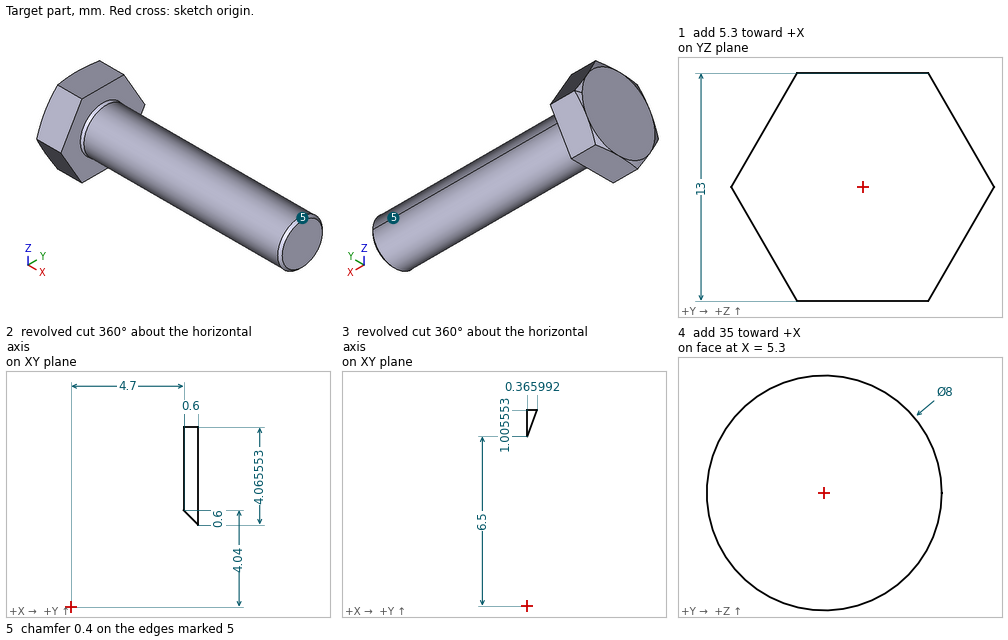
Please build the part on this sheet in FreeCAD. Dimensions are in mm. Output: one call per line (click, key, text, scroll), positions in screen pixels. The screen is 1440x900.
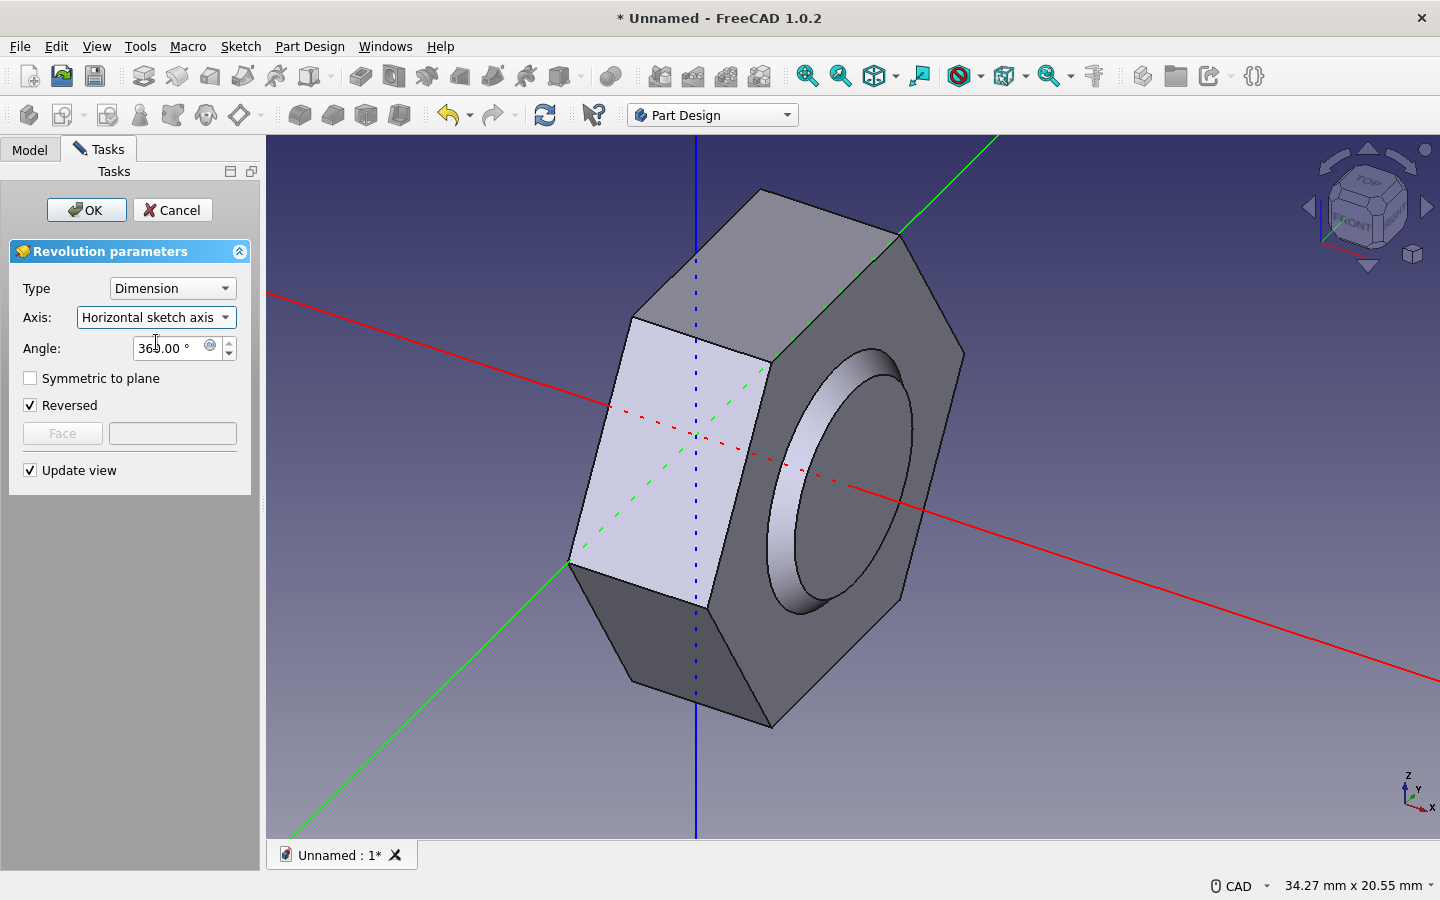
click(87, 210)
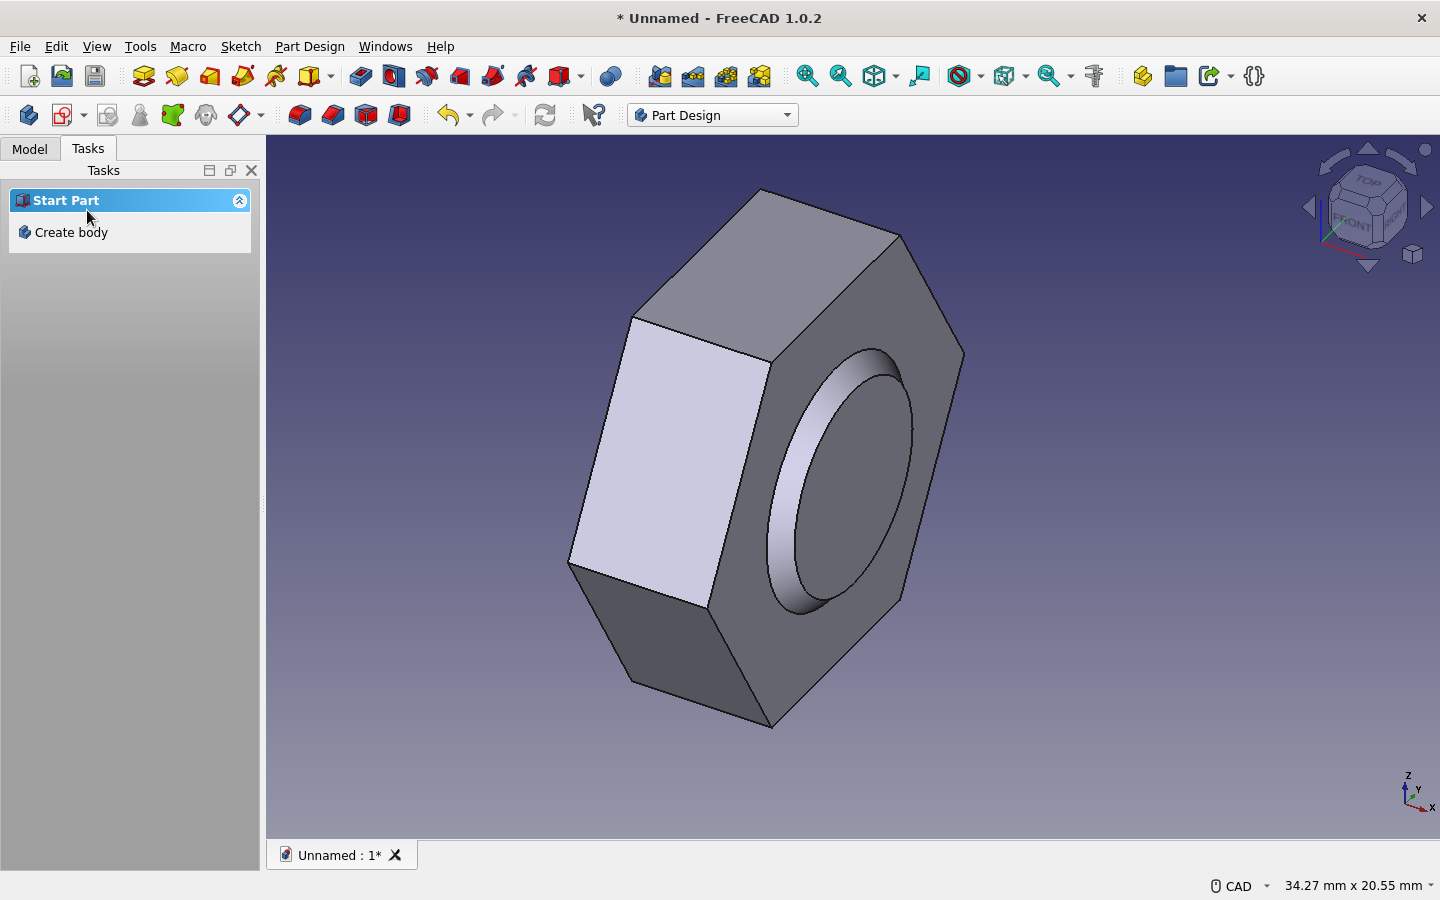
key(v)
key(f)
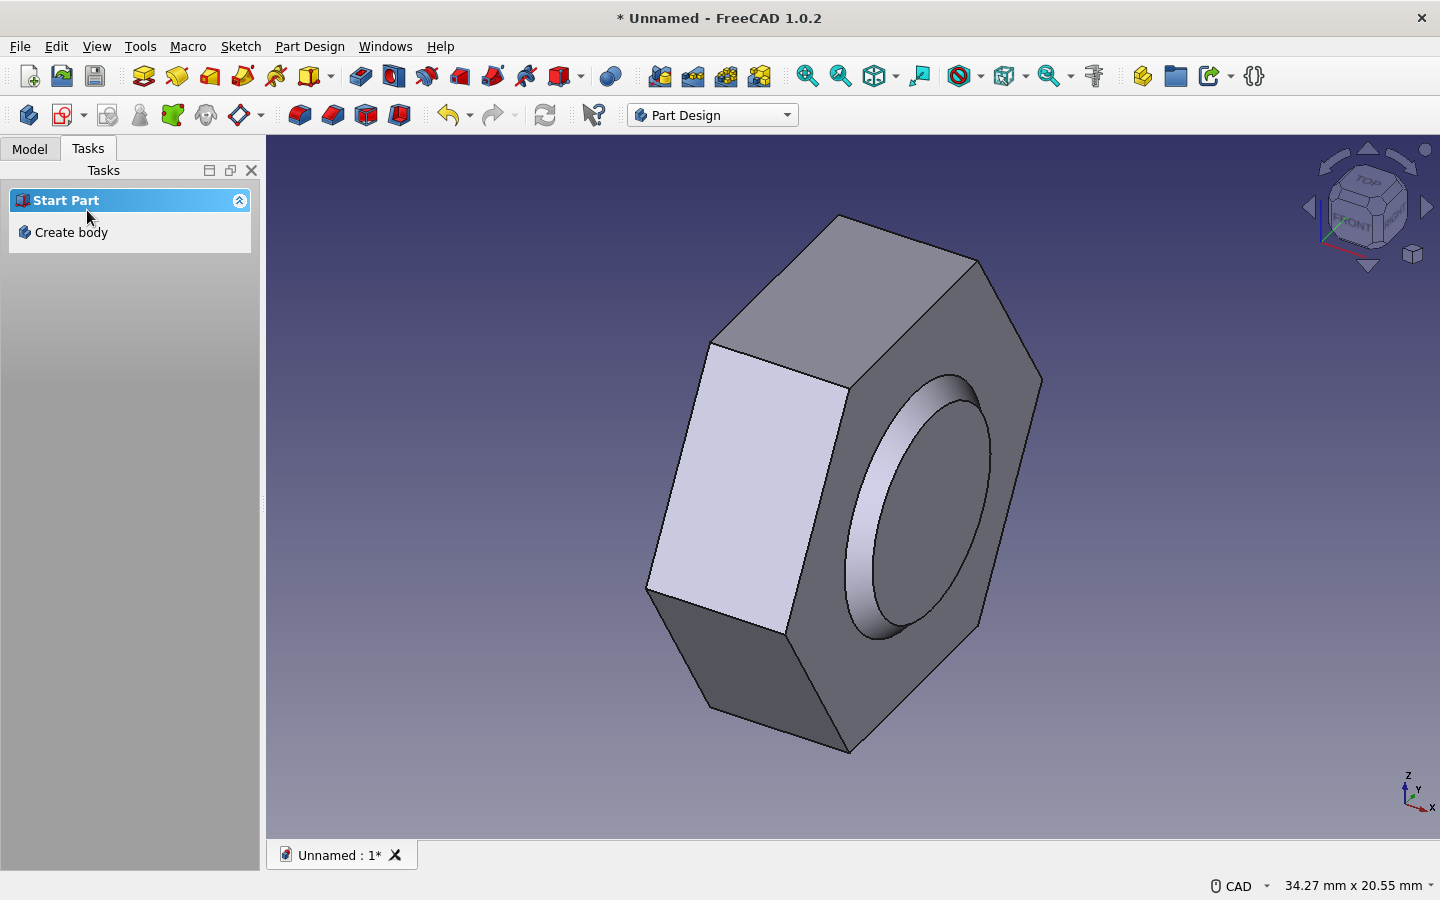
click(62, 116)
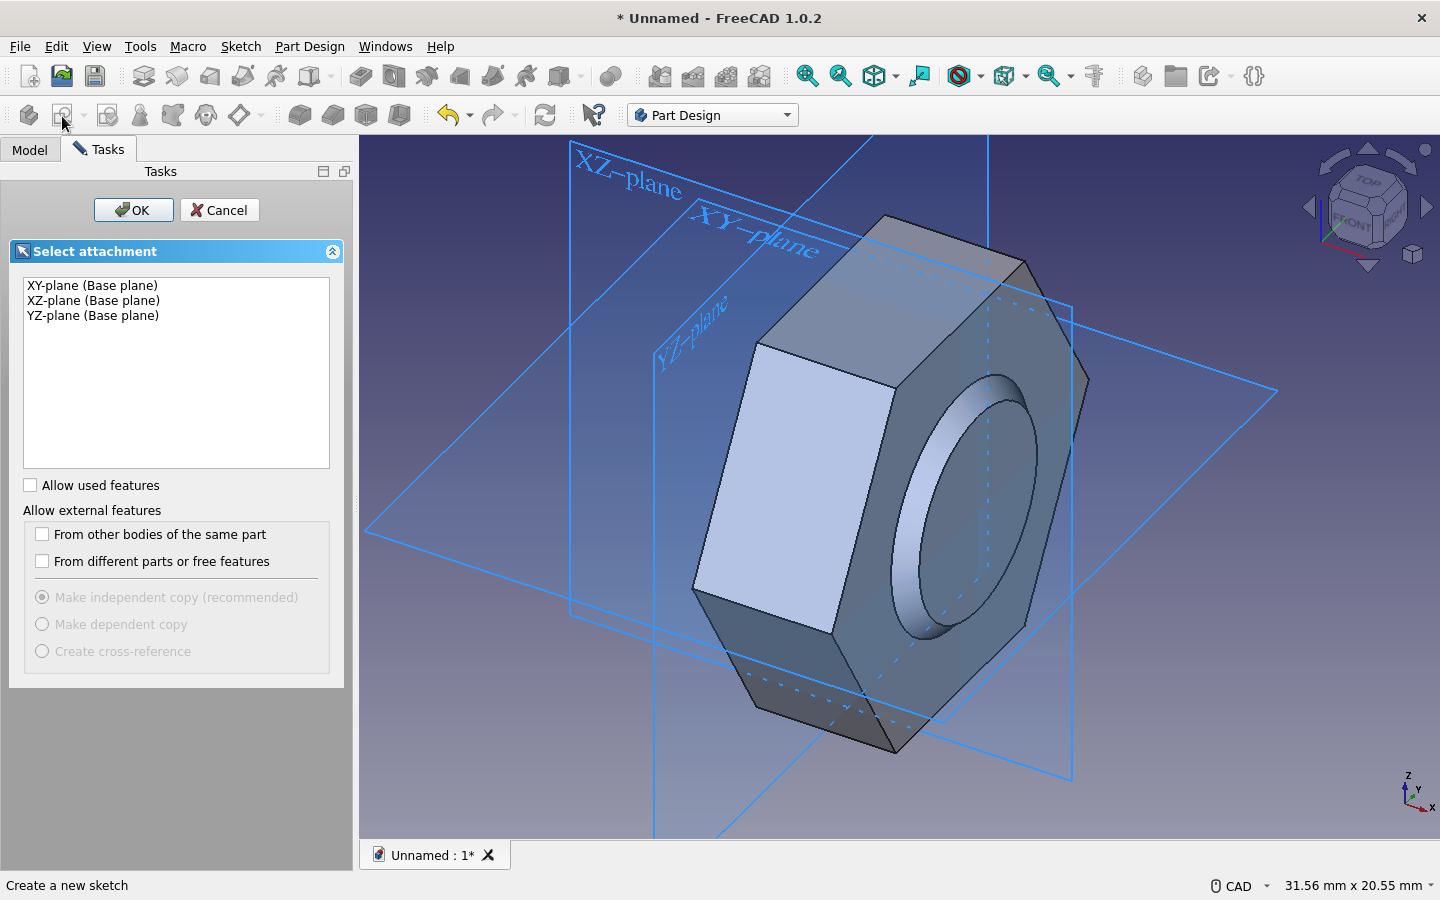
click(84, 286)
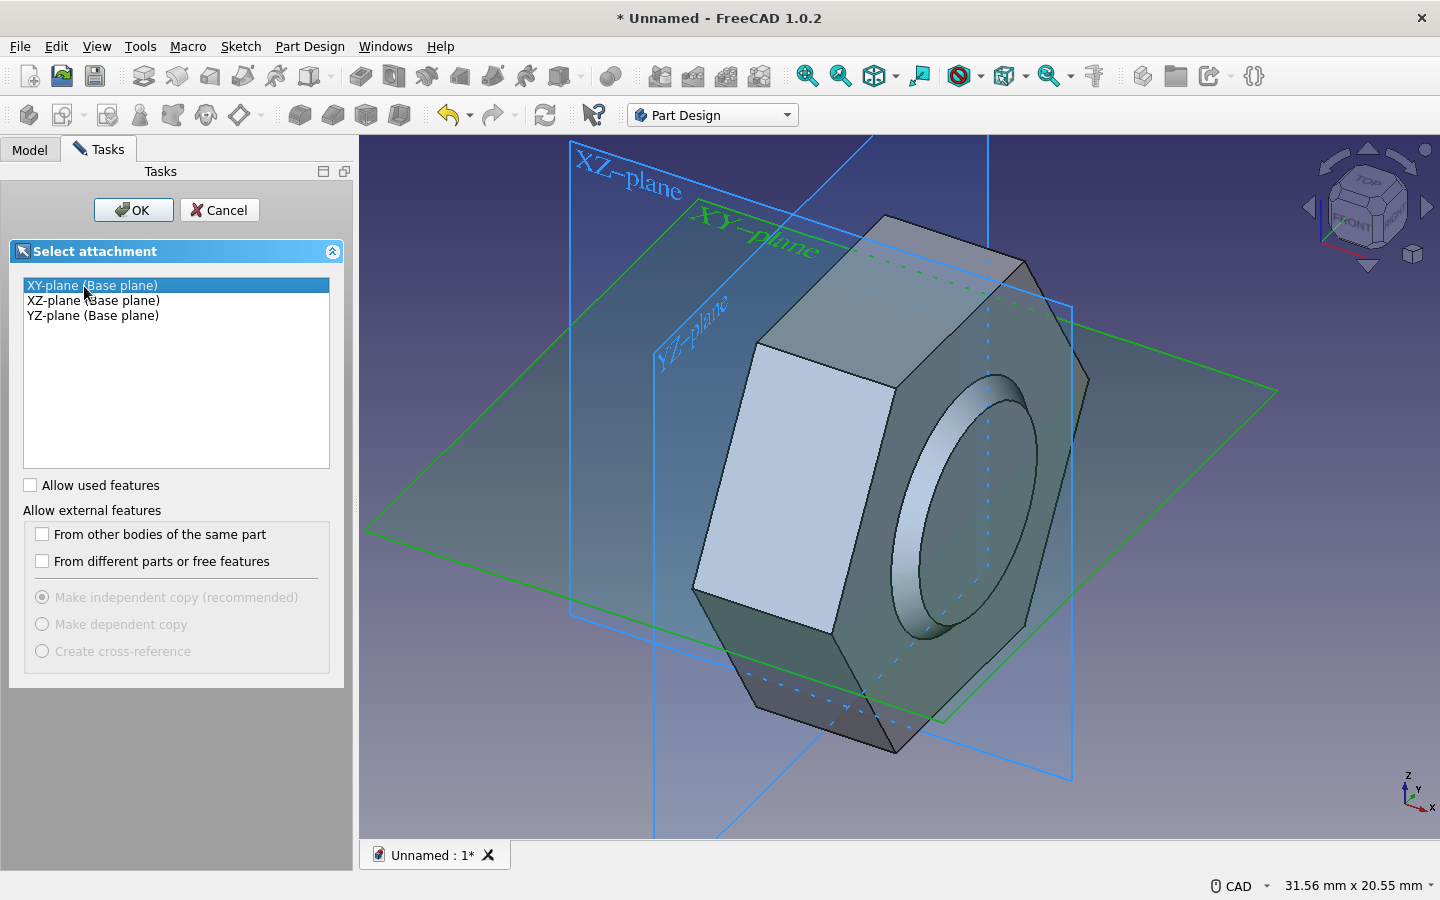
click(134, 210)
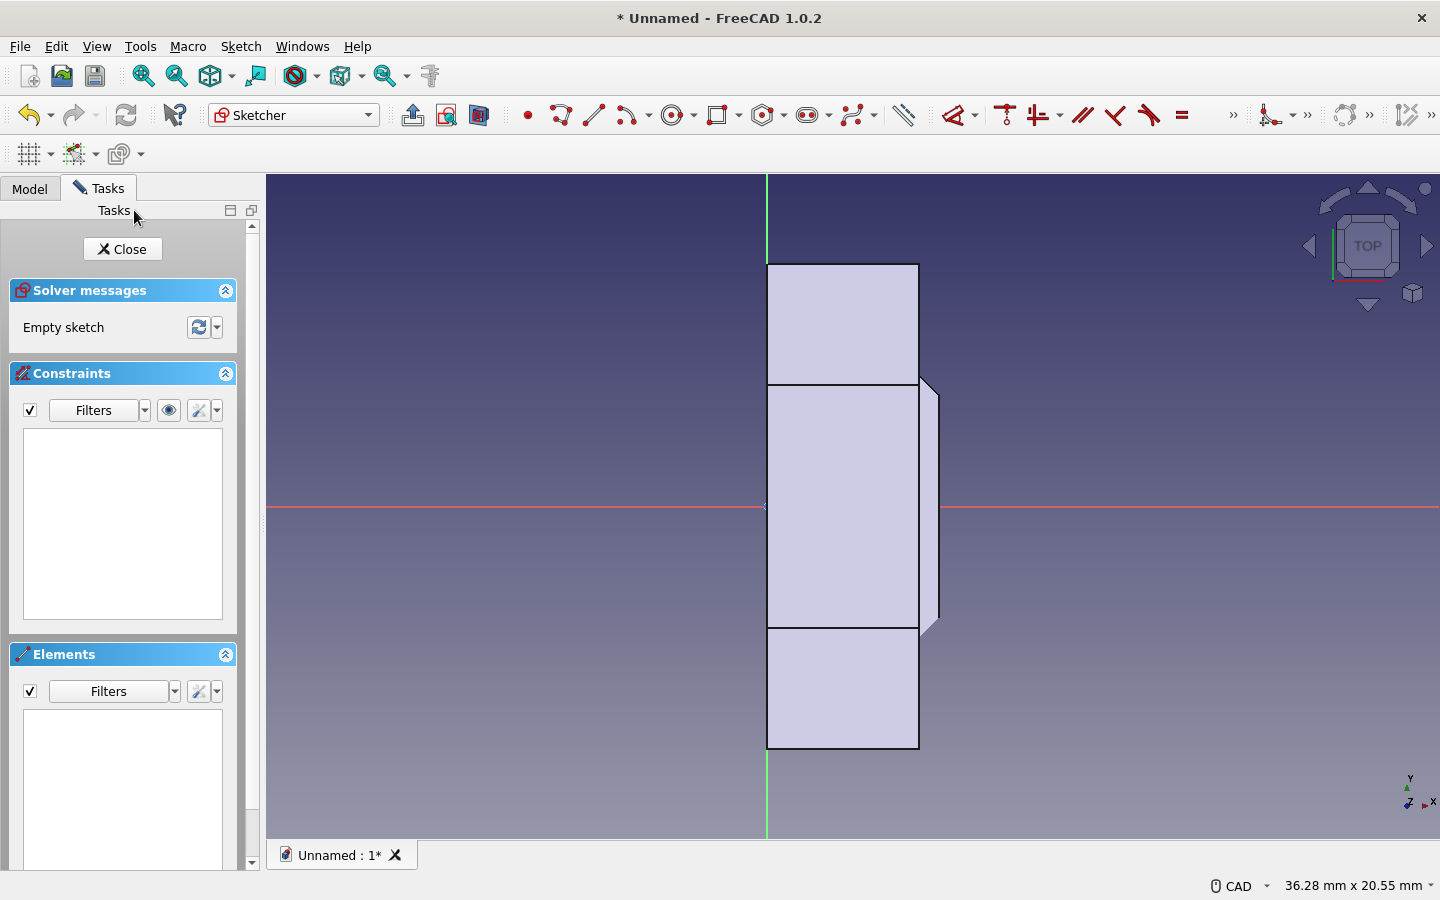
click(479, 116)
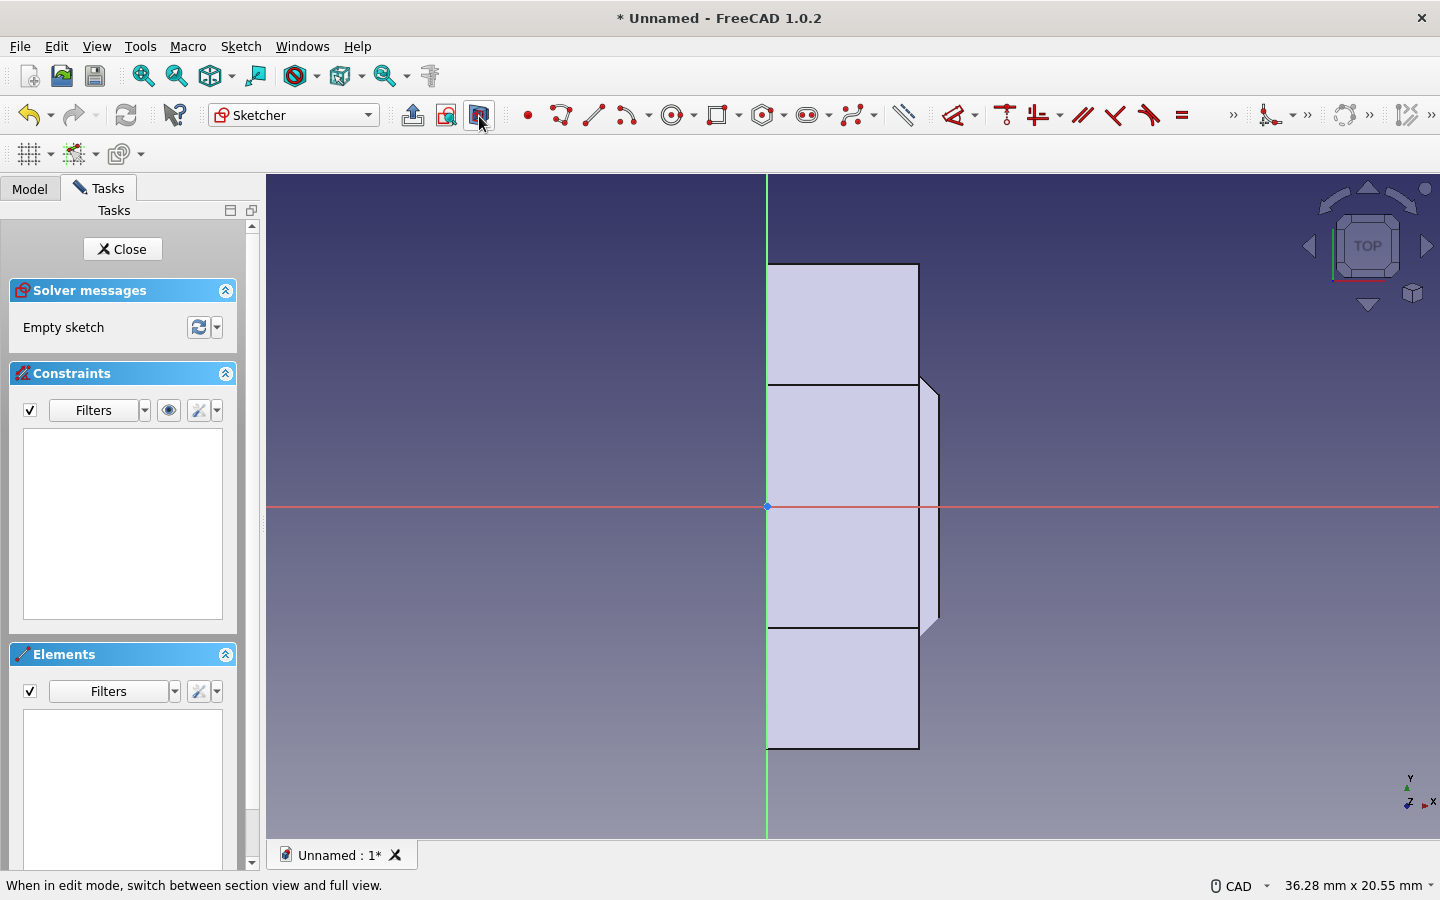
scroll(772, 262, up, 13)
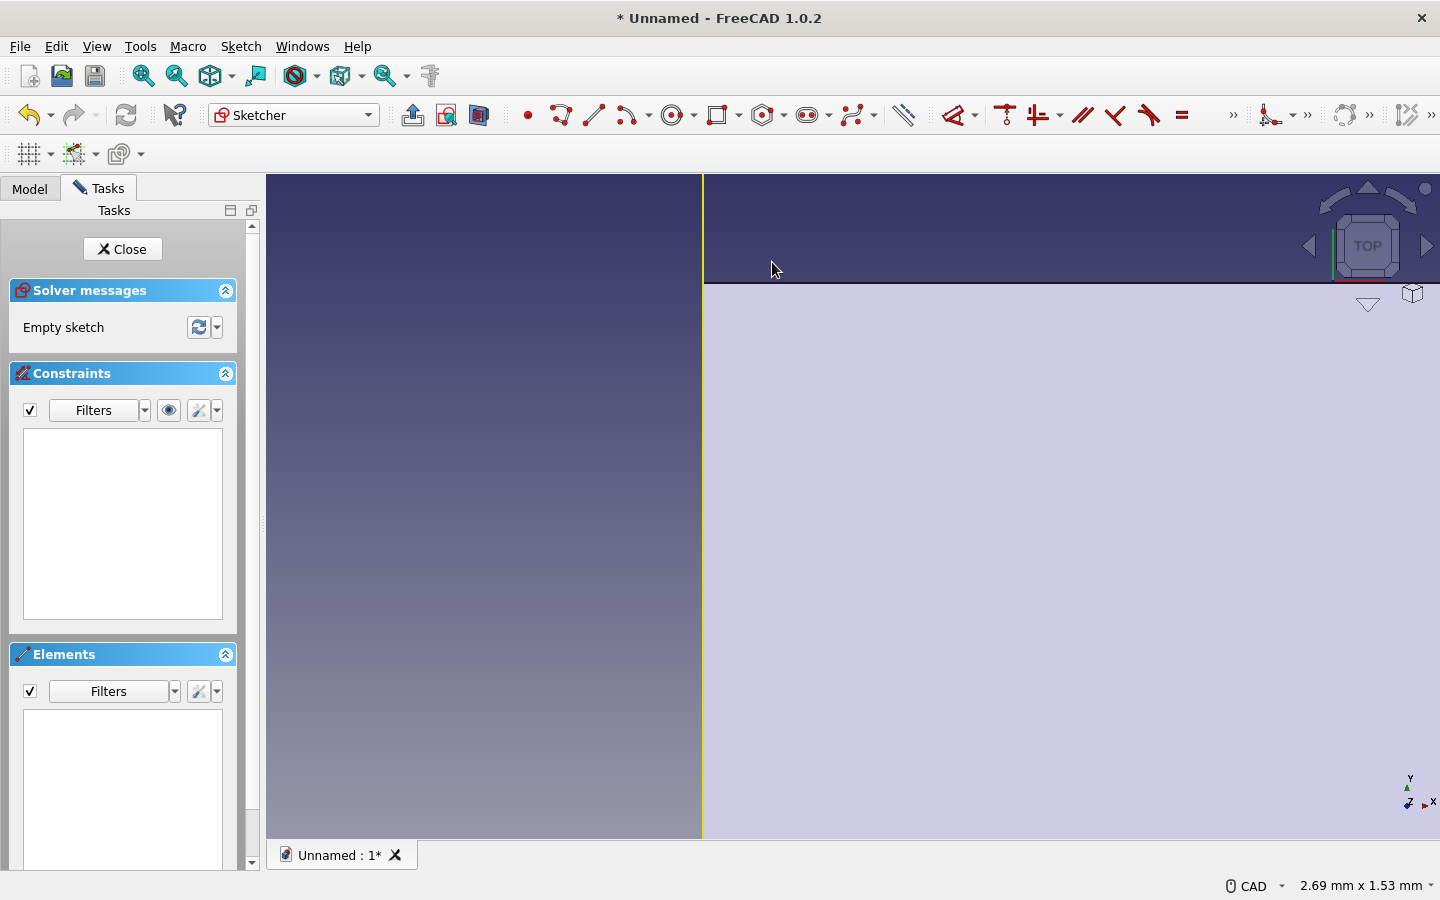
key(g)
key(m)